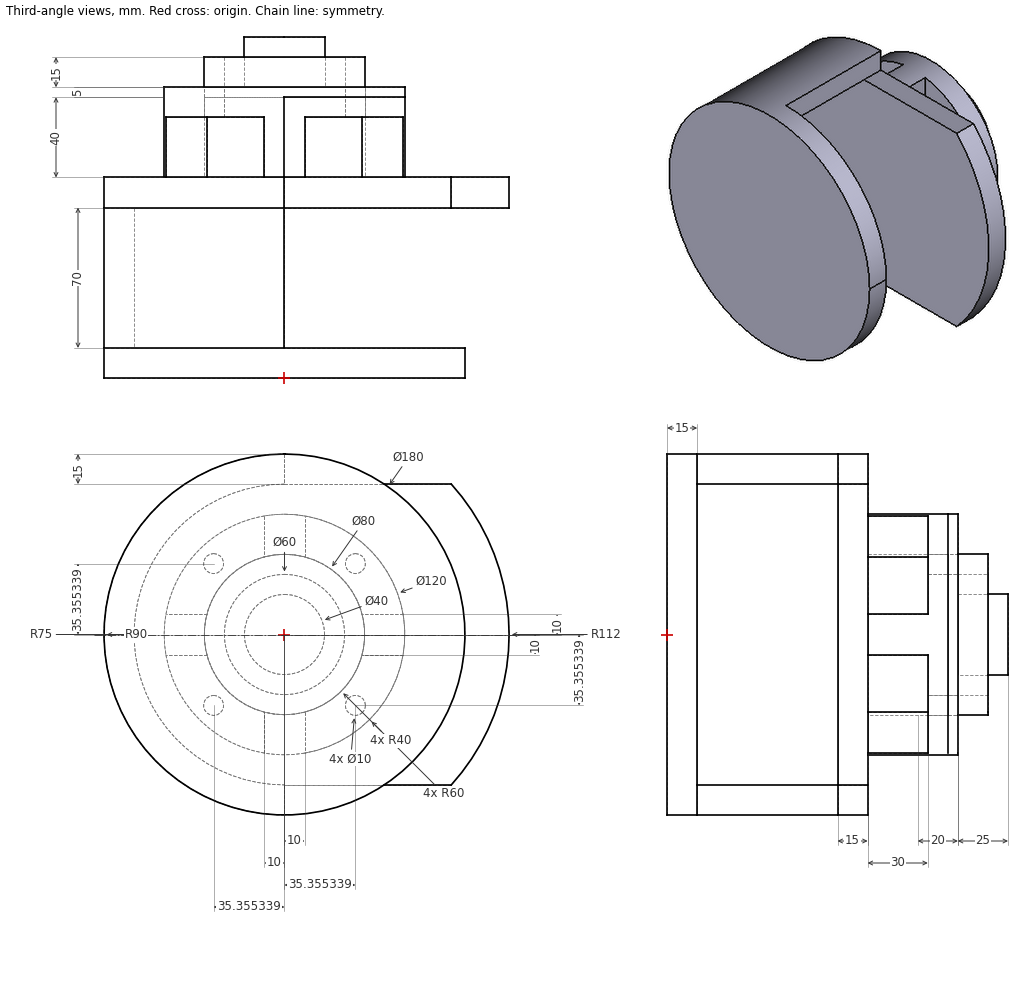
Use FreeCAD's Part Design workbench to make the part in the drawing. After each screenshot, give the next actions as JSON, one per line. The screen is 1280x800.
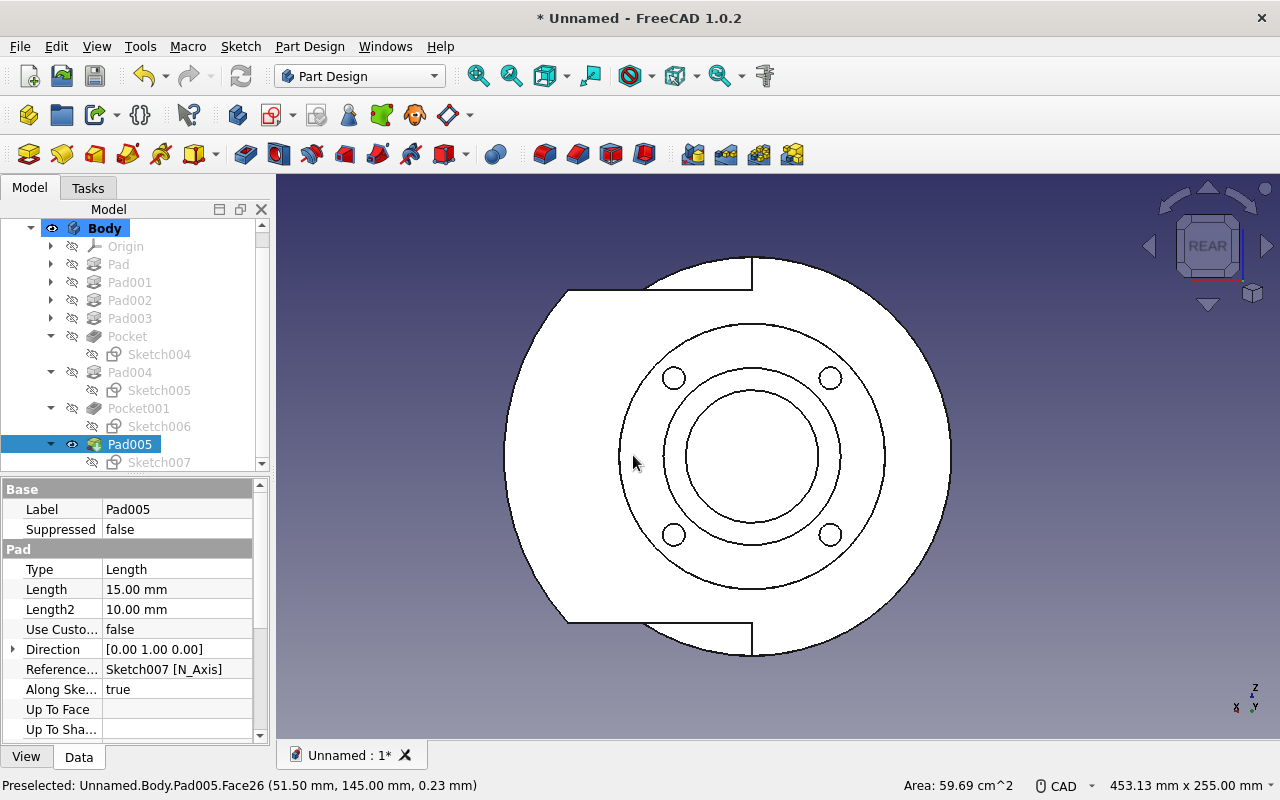
{"action": "left_click", "coordinate": [270, 116]}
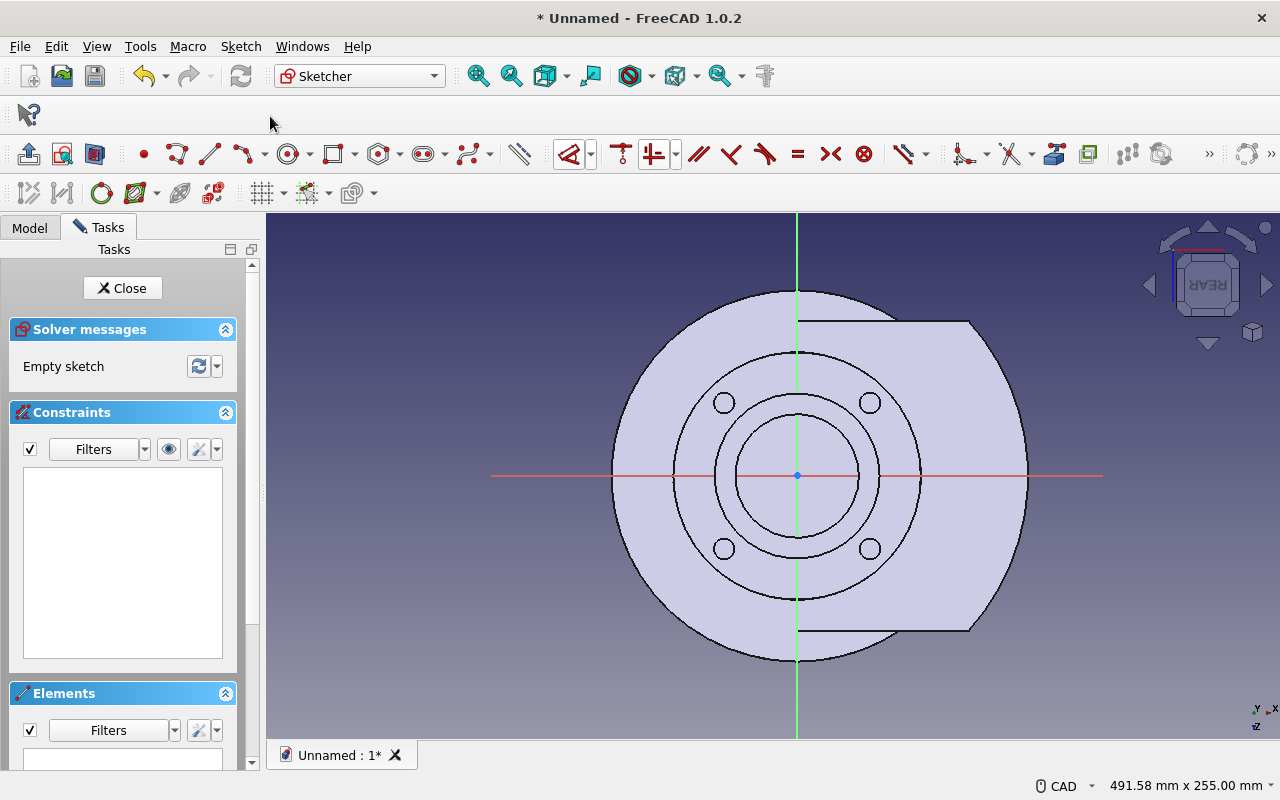
{"action": "scroll", "coordinate": [827, 476], "scroll_direction": "up", "scroll_amount": 7}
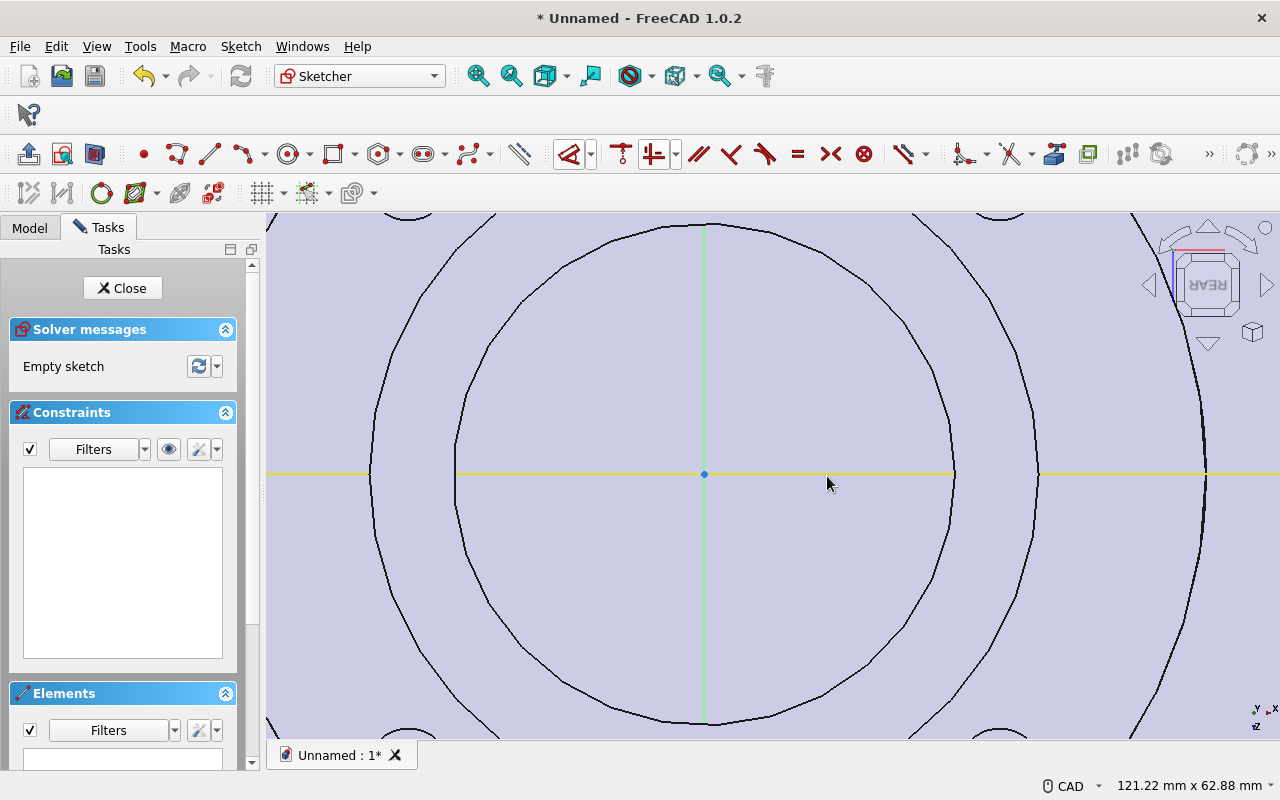
{"action": "key", "text": "g c"}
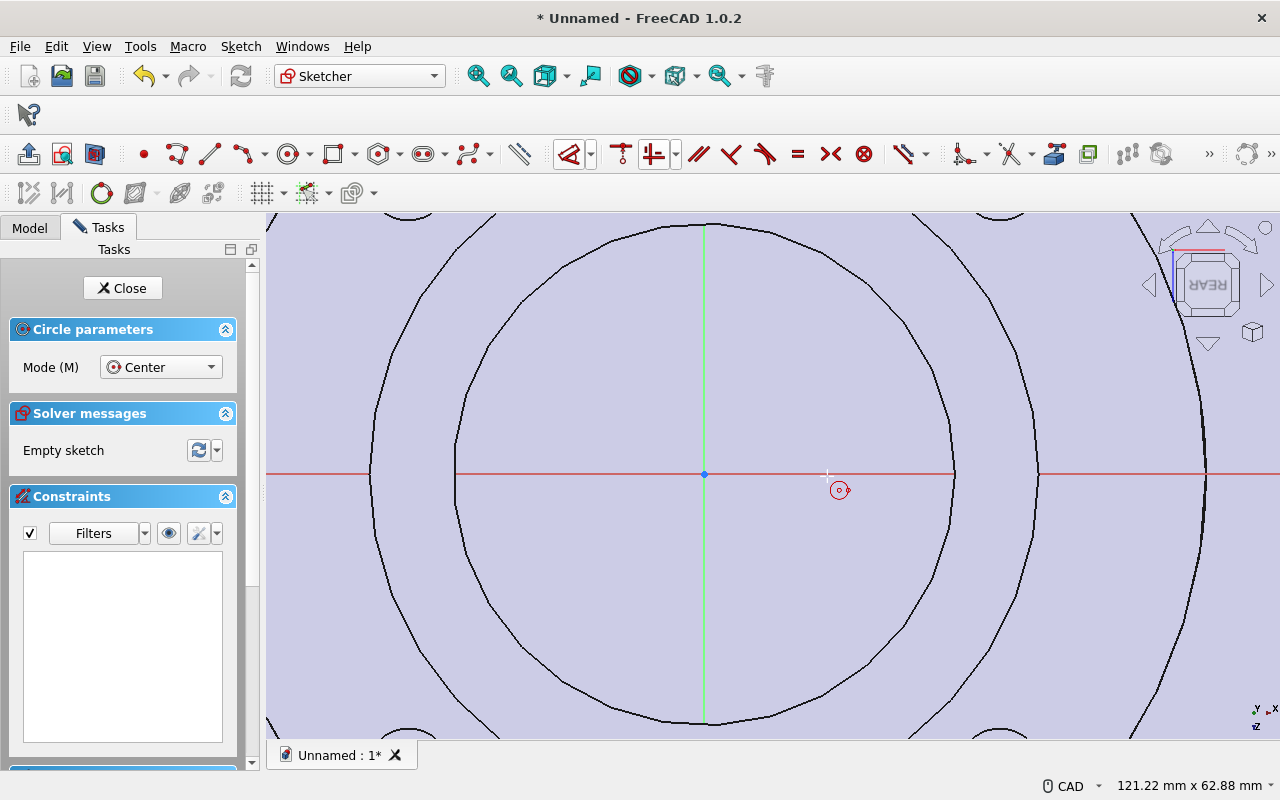
{"action": "left_click", "coordinate": [704, 474]}
{"action": "left_click", "coordinate": [822, 356]}
{"action": "key", "text": "Escape"}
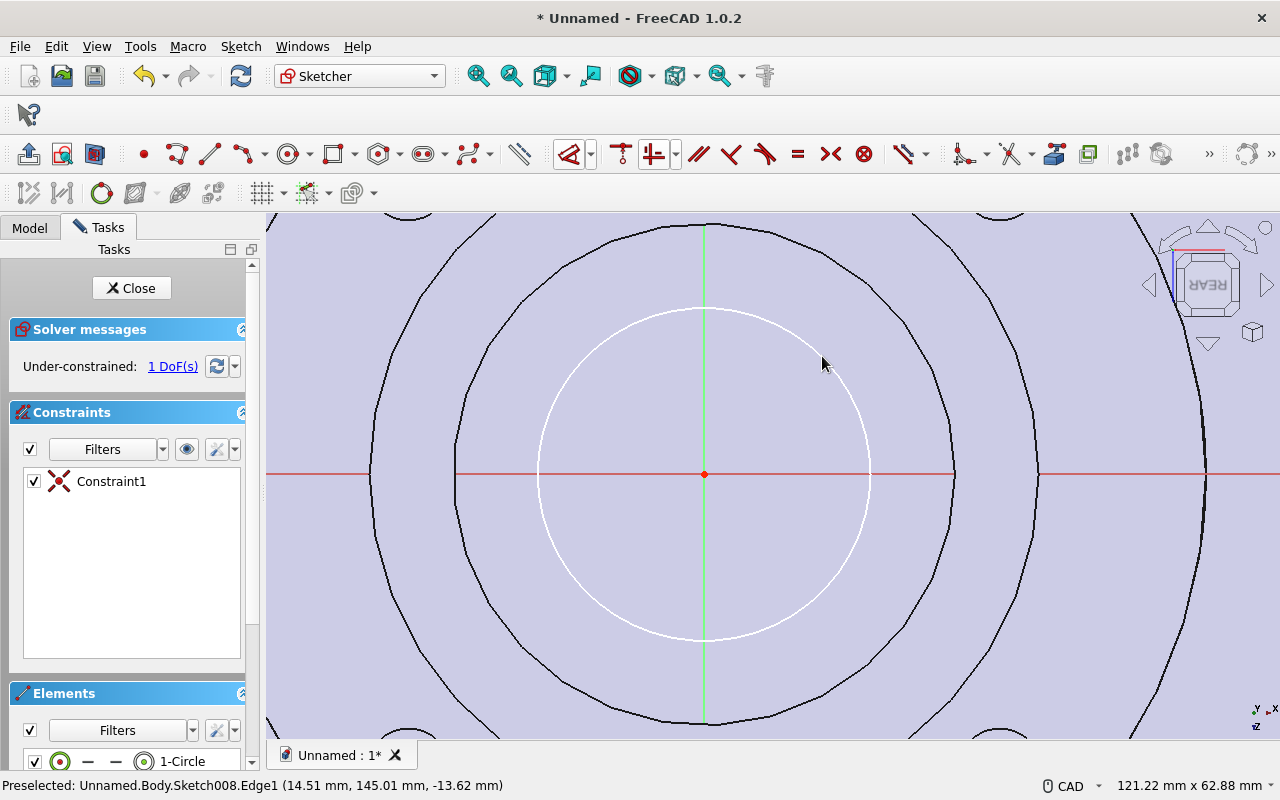
{"action": "left_click", "coordinate": [821, 356]}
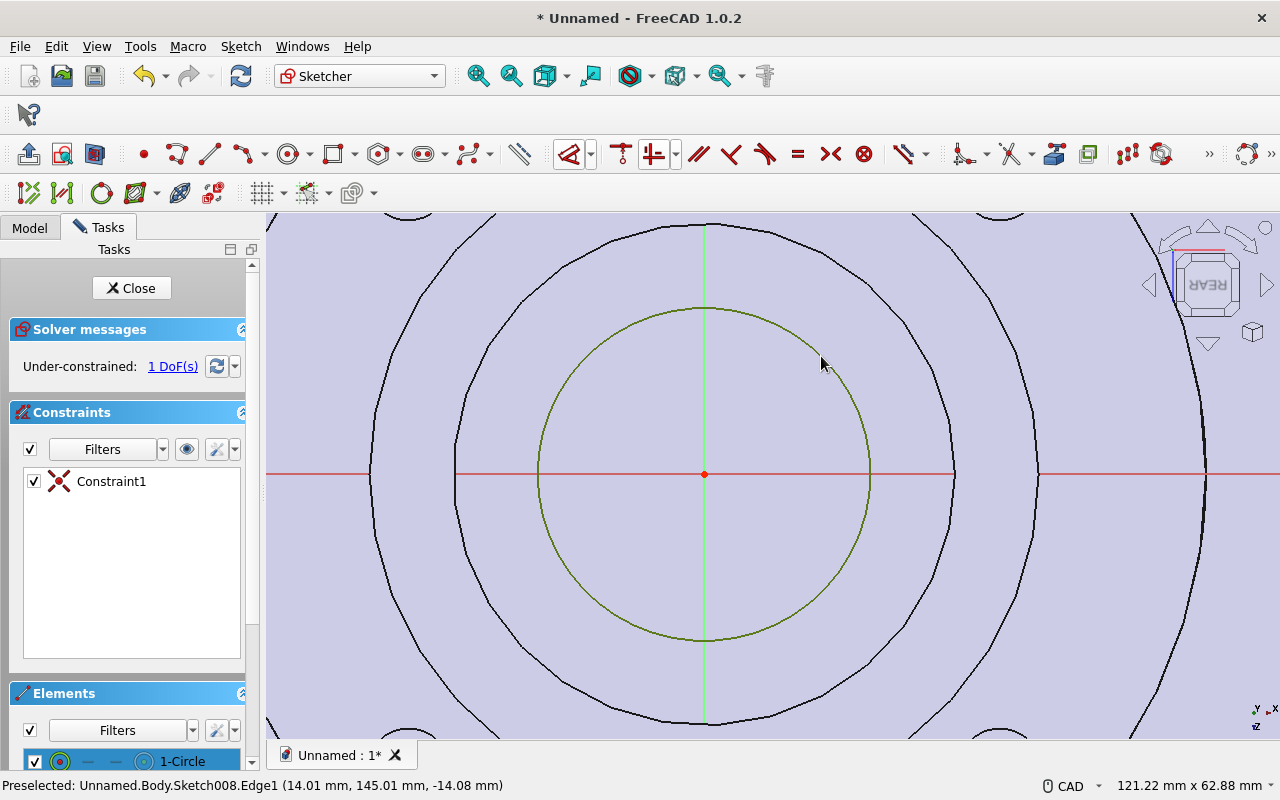
{"action": "left_click", "coordinate": [590, 154]}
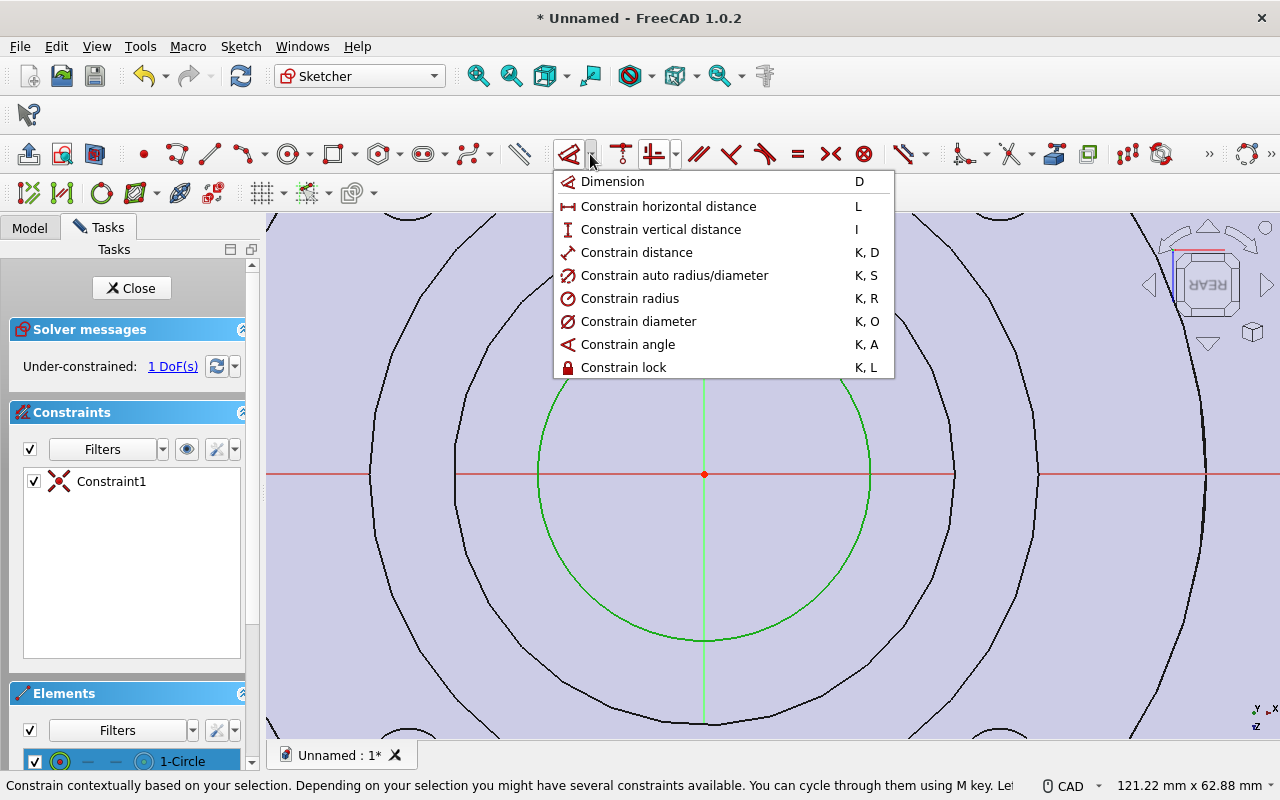
{"action": "left_click", "coordinate": [724, 322]}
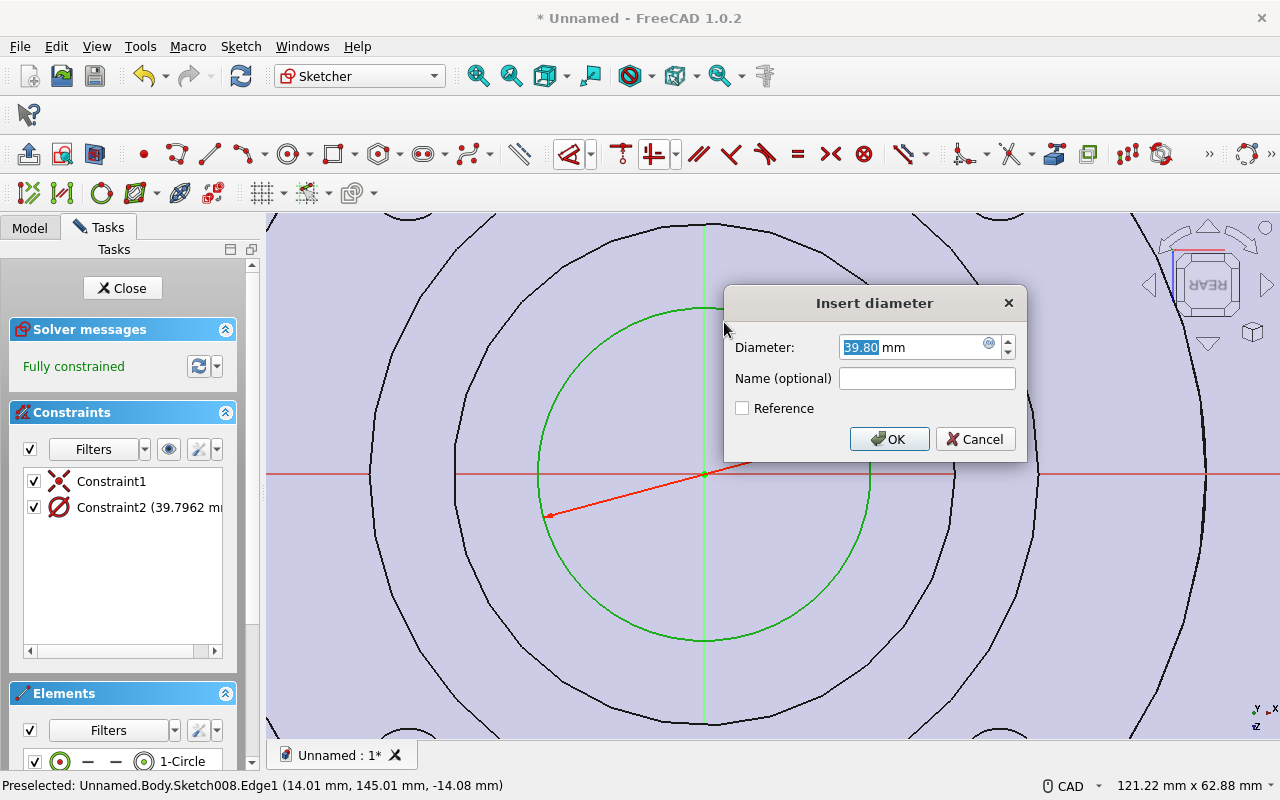
{"action": "type", "text": "40"}
{"action": "key", "text": "Return"}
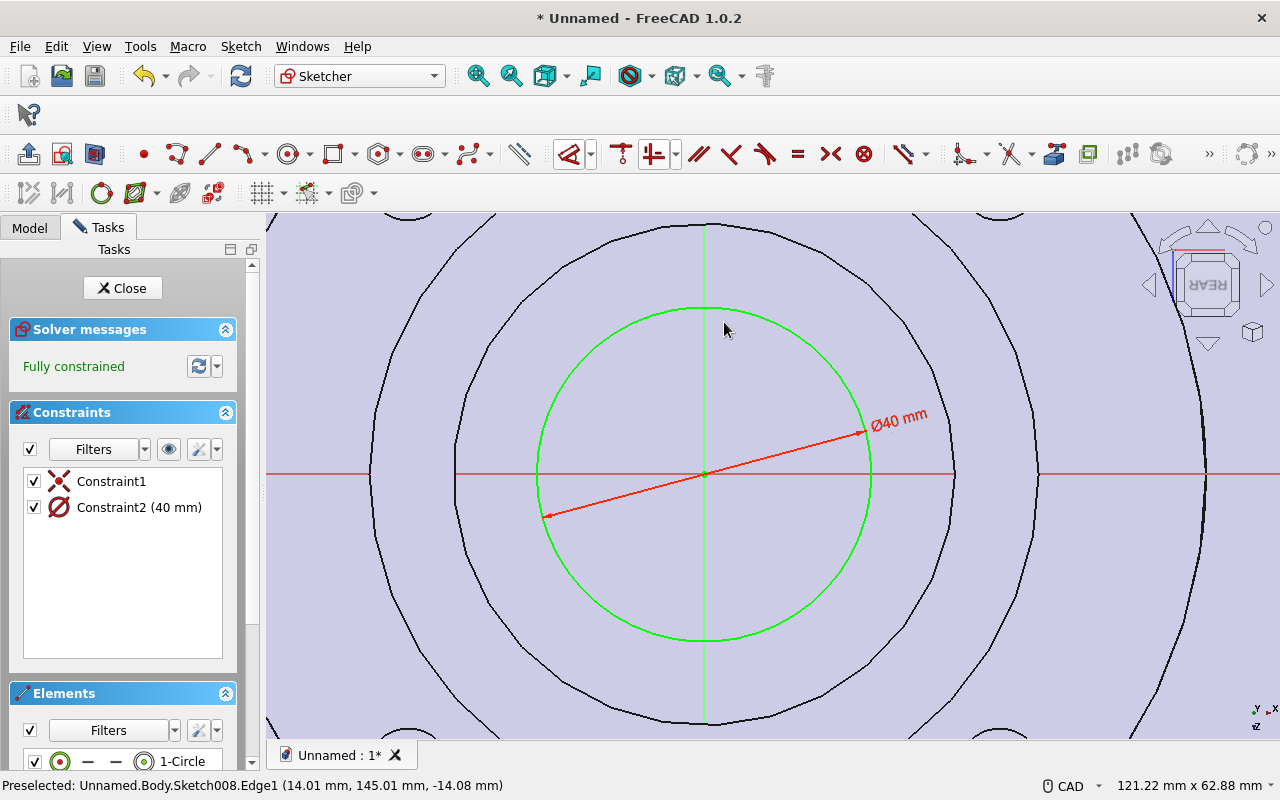
{"action": "left_click", "coordinate": [123, 288]}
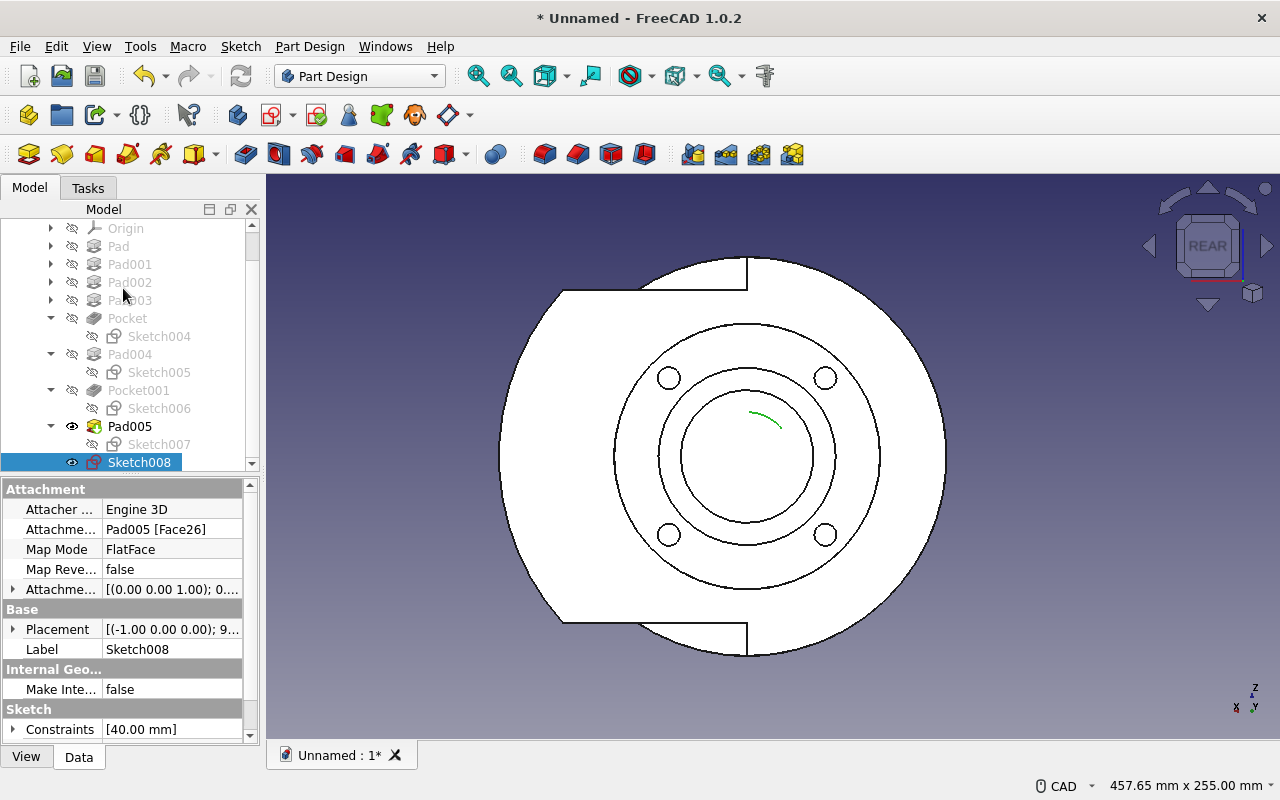
{"action": "left_click", "coordinate": [29, 154]}